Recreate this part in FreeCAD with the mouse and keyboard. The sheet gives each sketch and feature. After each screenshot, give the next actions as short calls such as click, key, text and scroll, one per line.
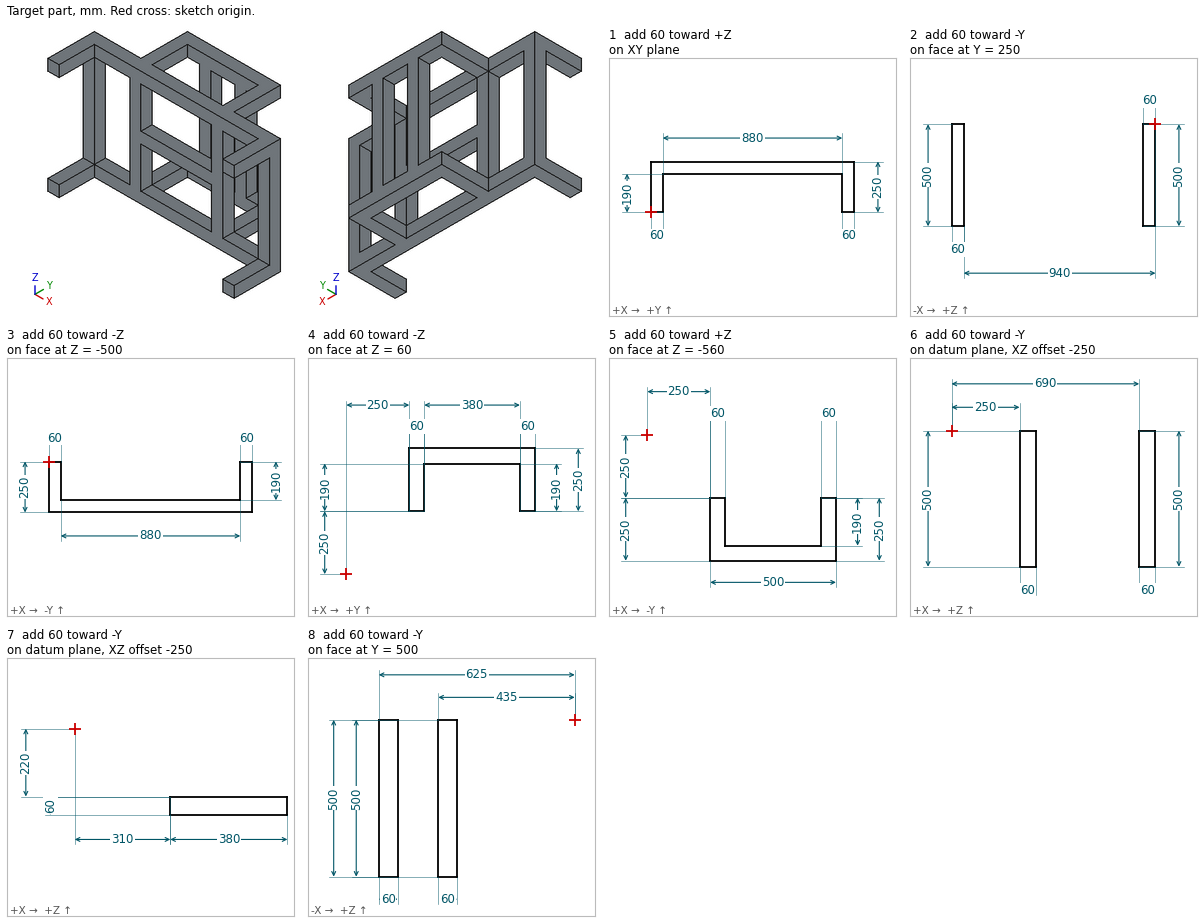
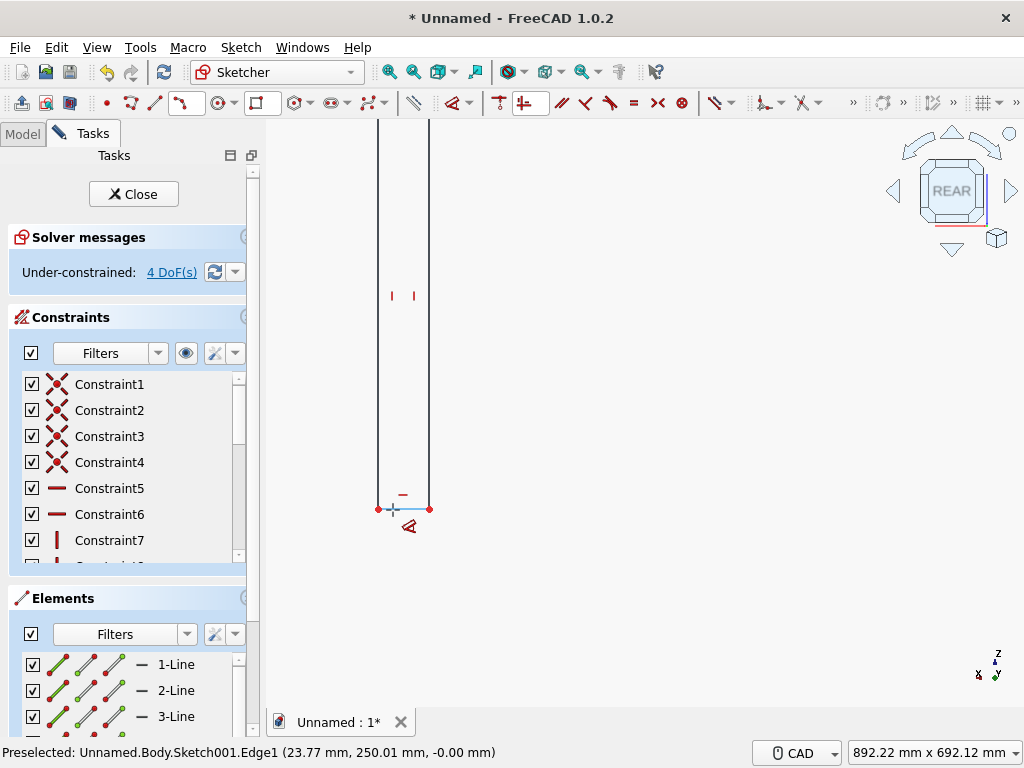
click(394, 509)
click(404, 543)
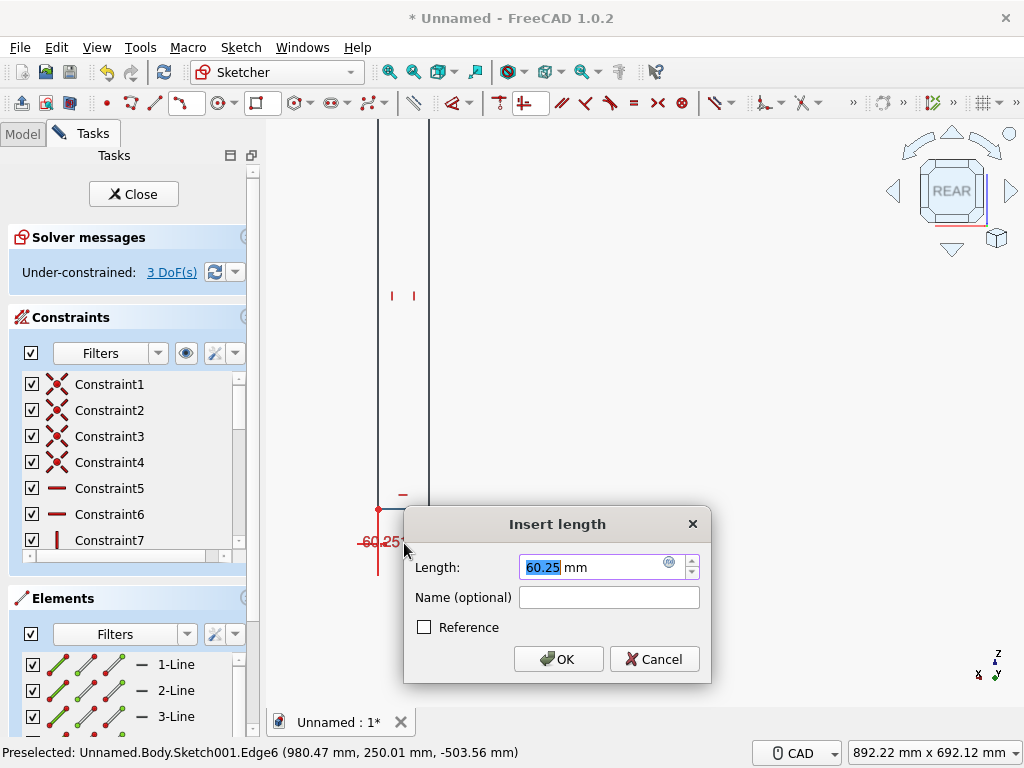
text(60)
key(Return)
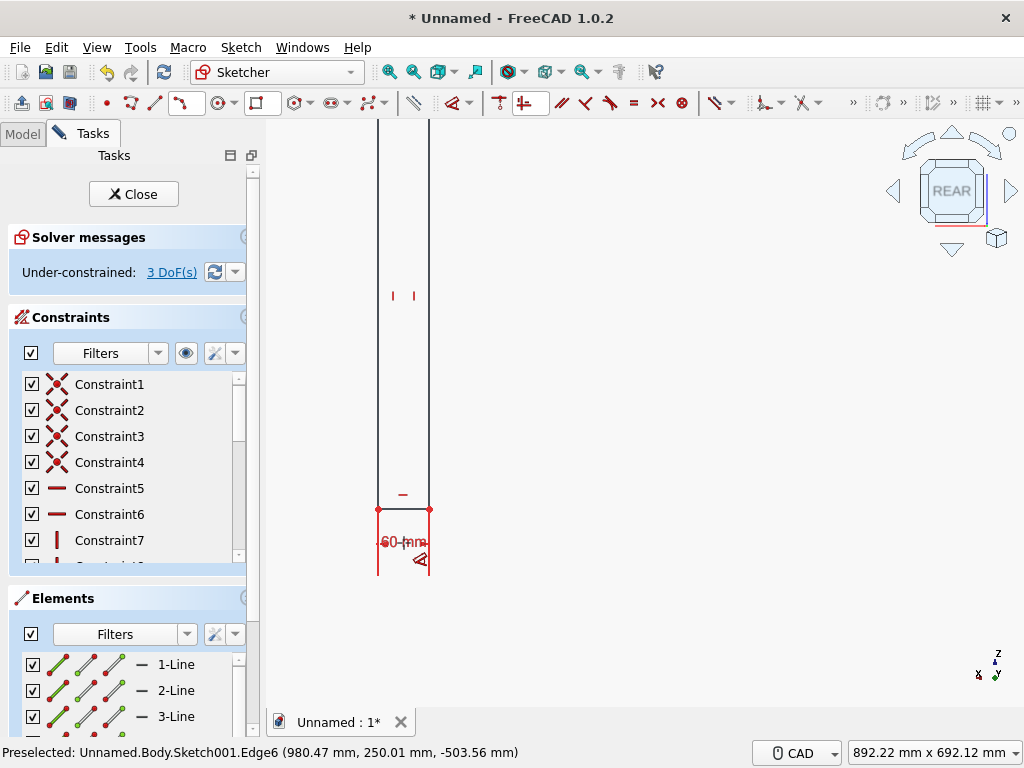
scroll(392, 510, down, 4)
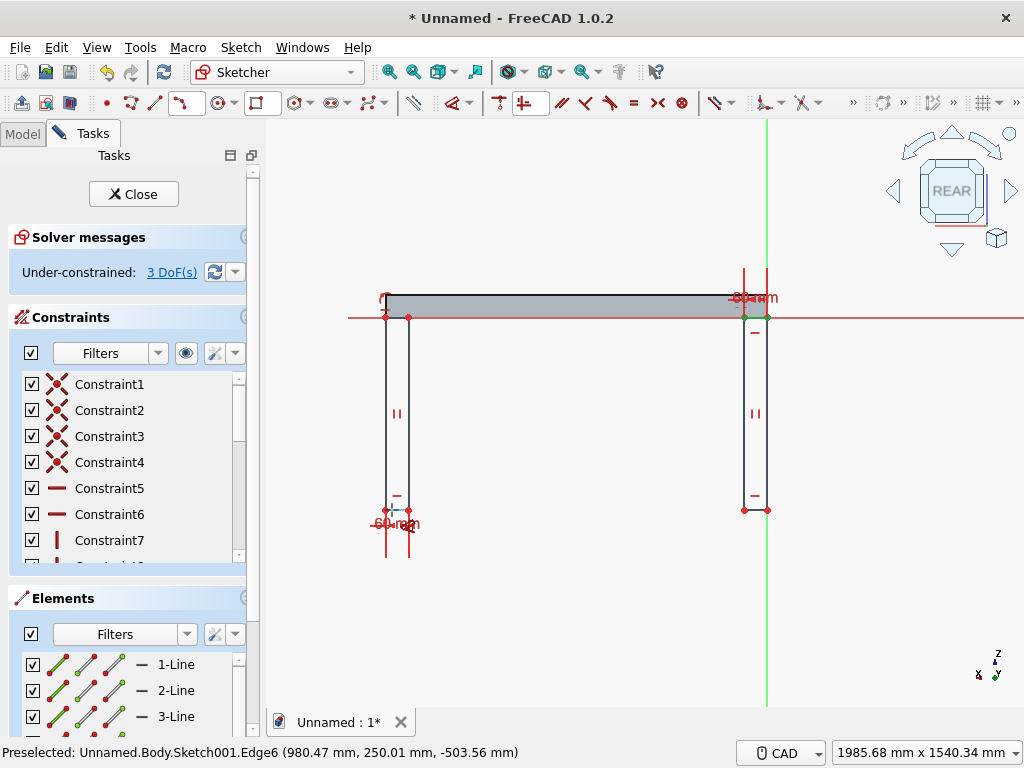
click(744, 375)
click(710, 414)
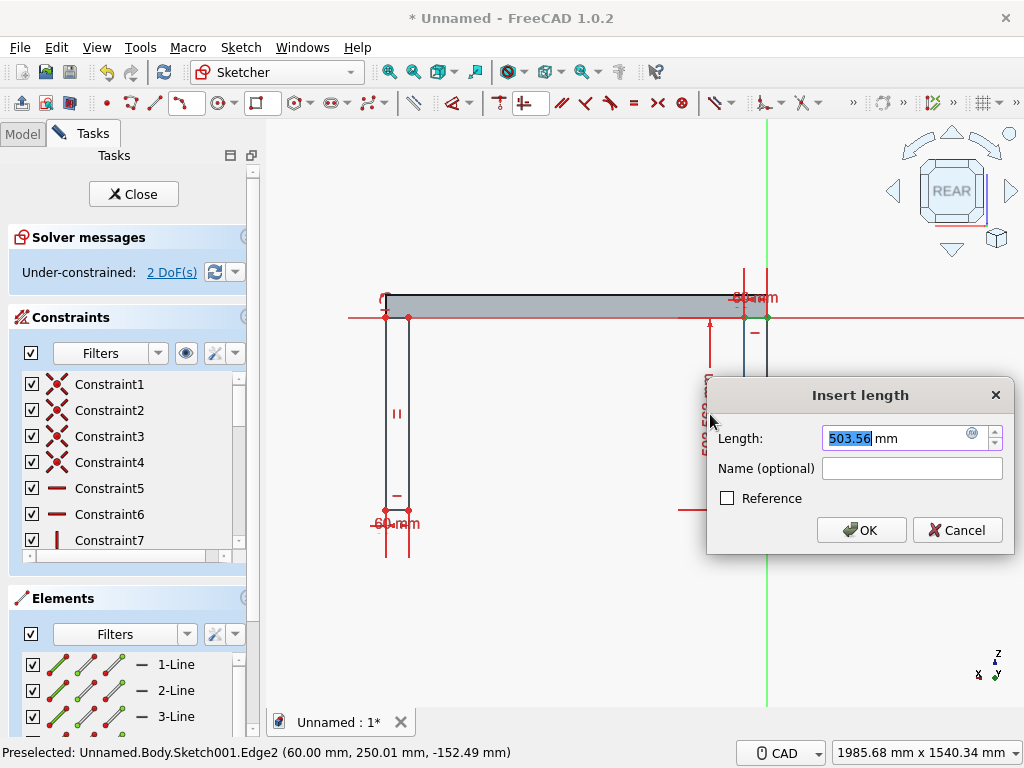
text(500)
key(Return)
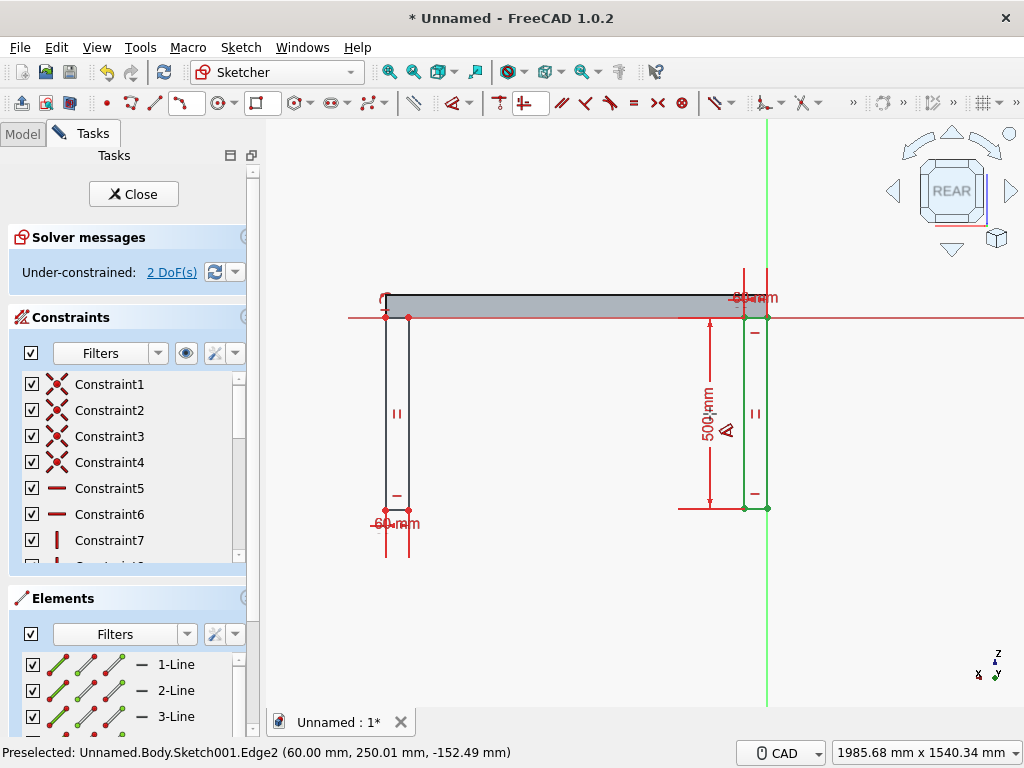
click(386, 375)
click(352, 414)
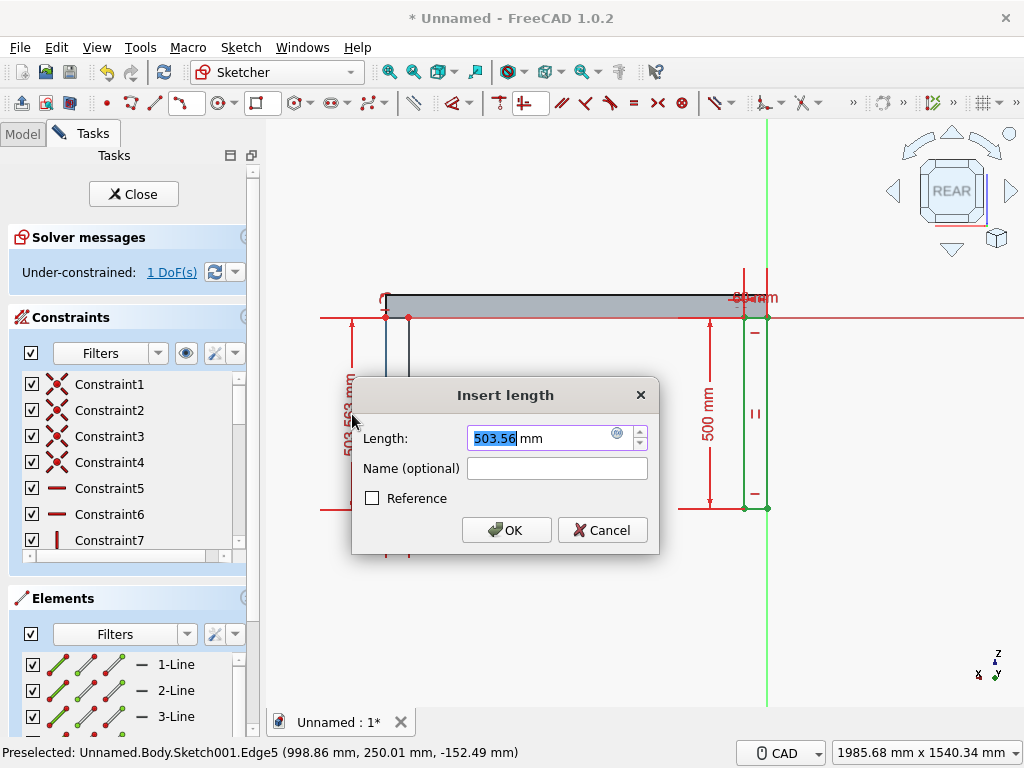
text(500)
key(Return)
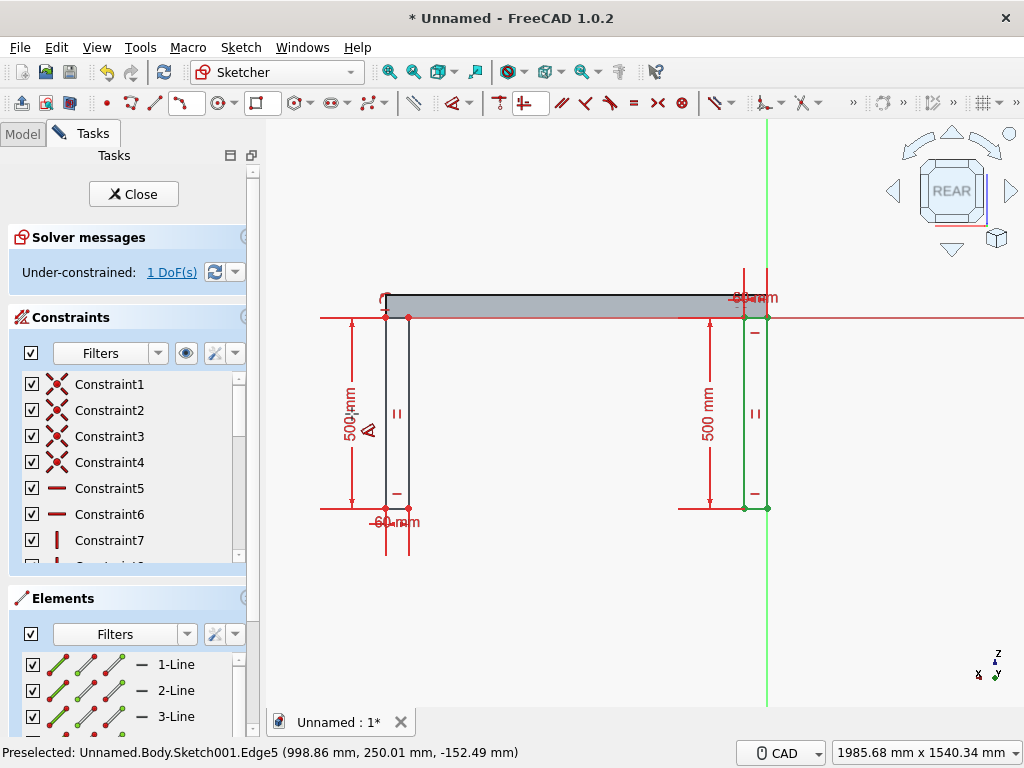
click(409, 509)
click(588, 543)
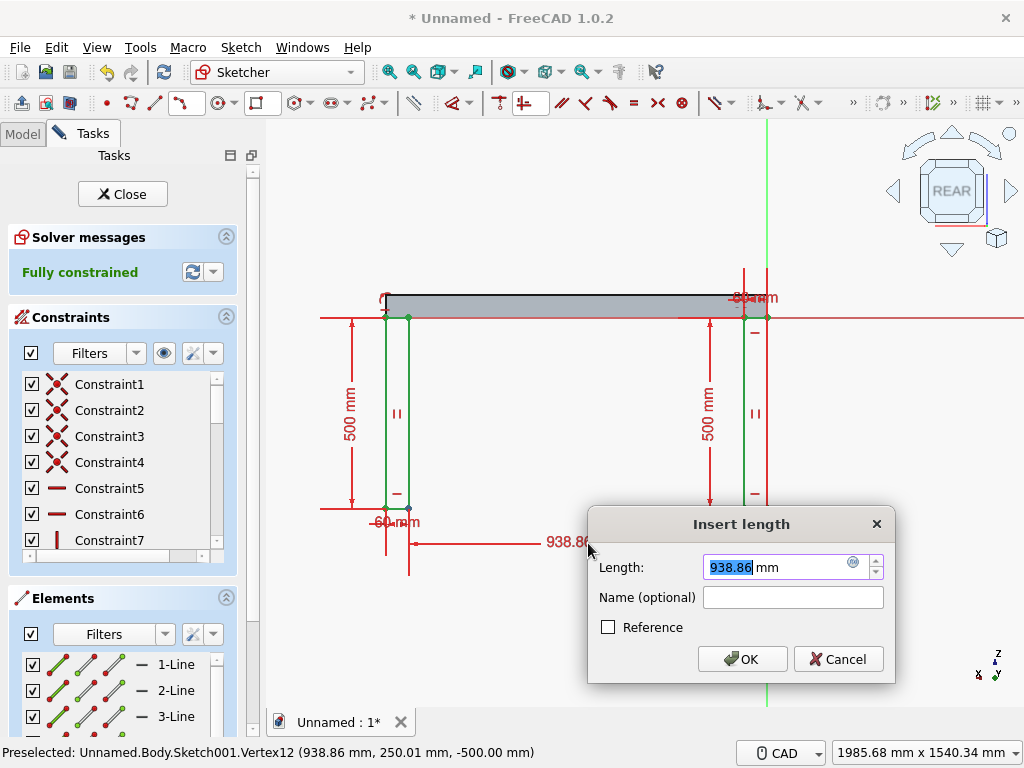
text(940)
key(Return)
key(Escape)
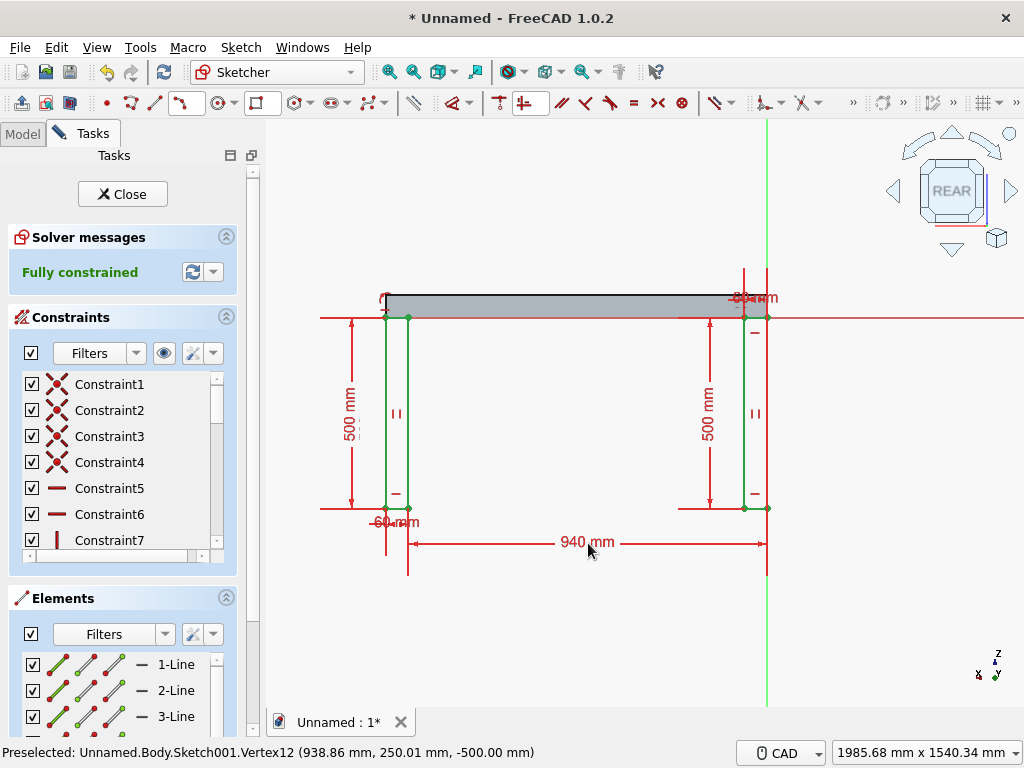
click(123, 194)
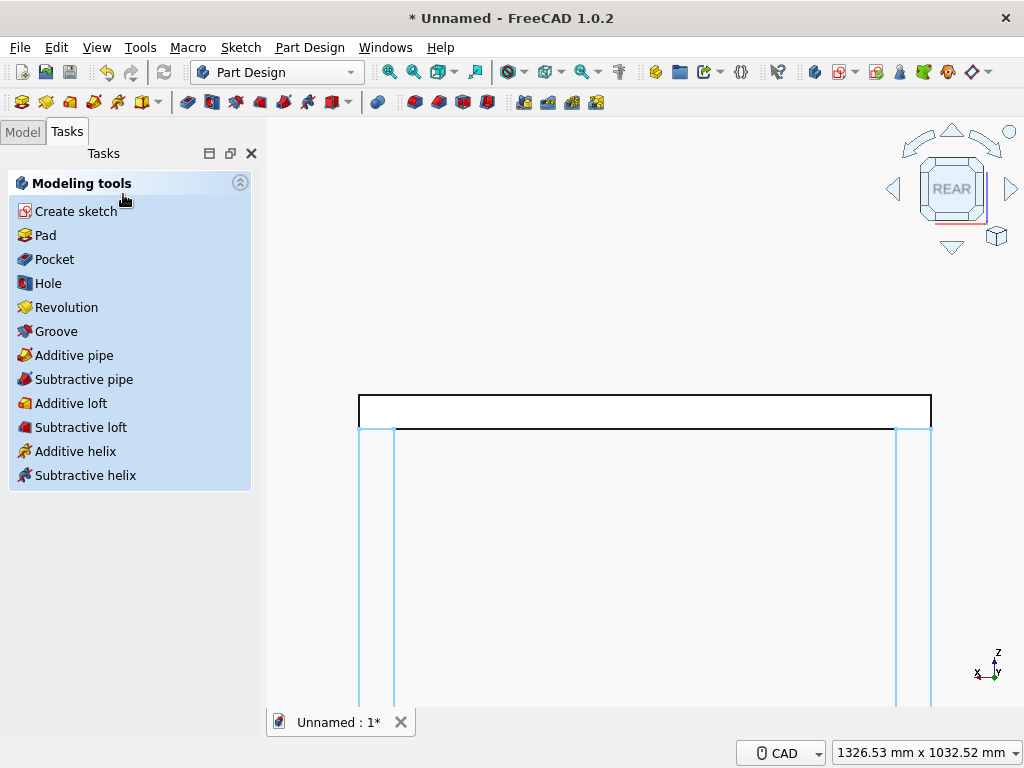
click(22, 102)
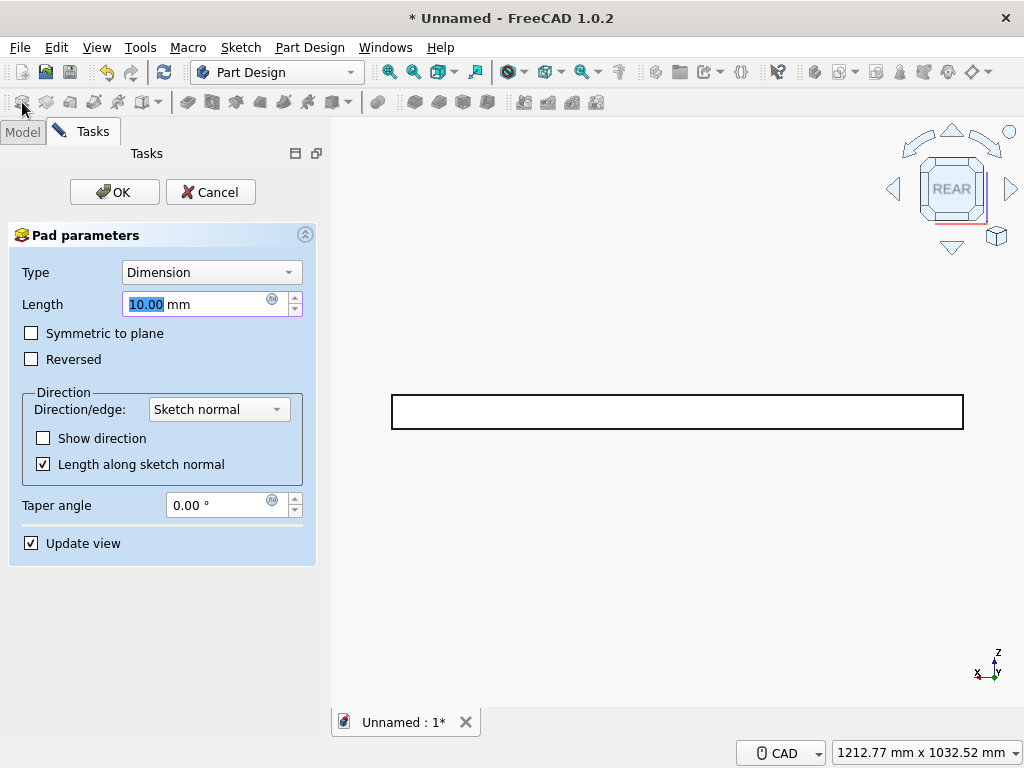
text(60)
key(Tab)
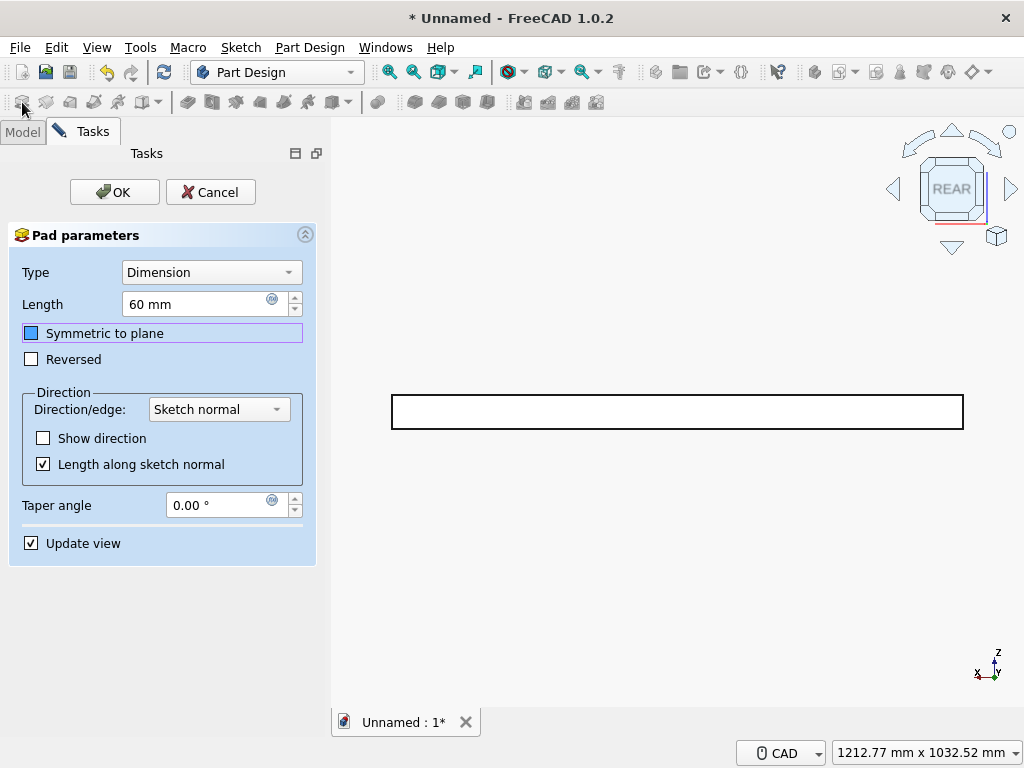
click(30, 359)